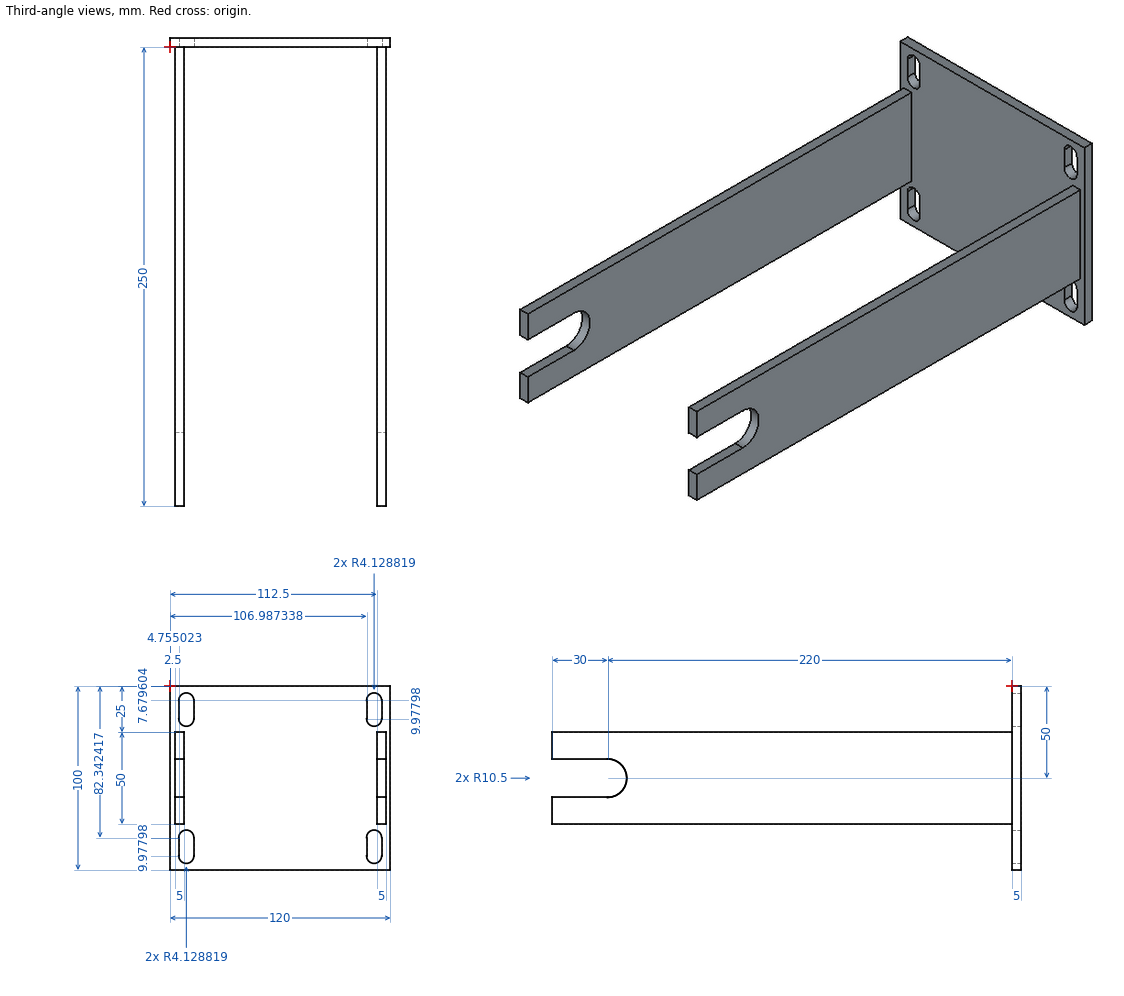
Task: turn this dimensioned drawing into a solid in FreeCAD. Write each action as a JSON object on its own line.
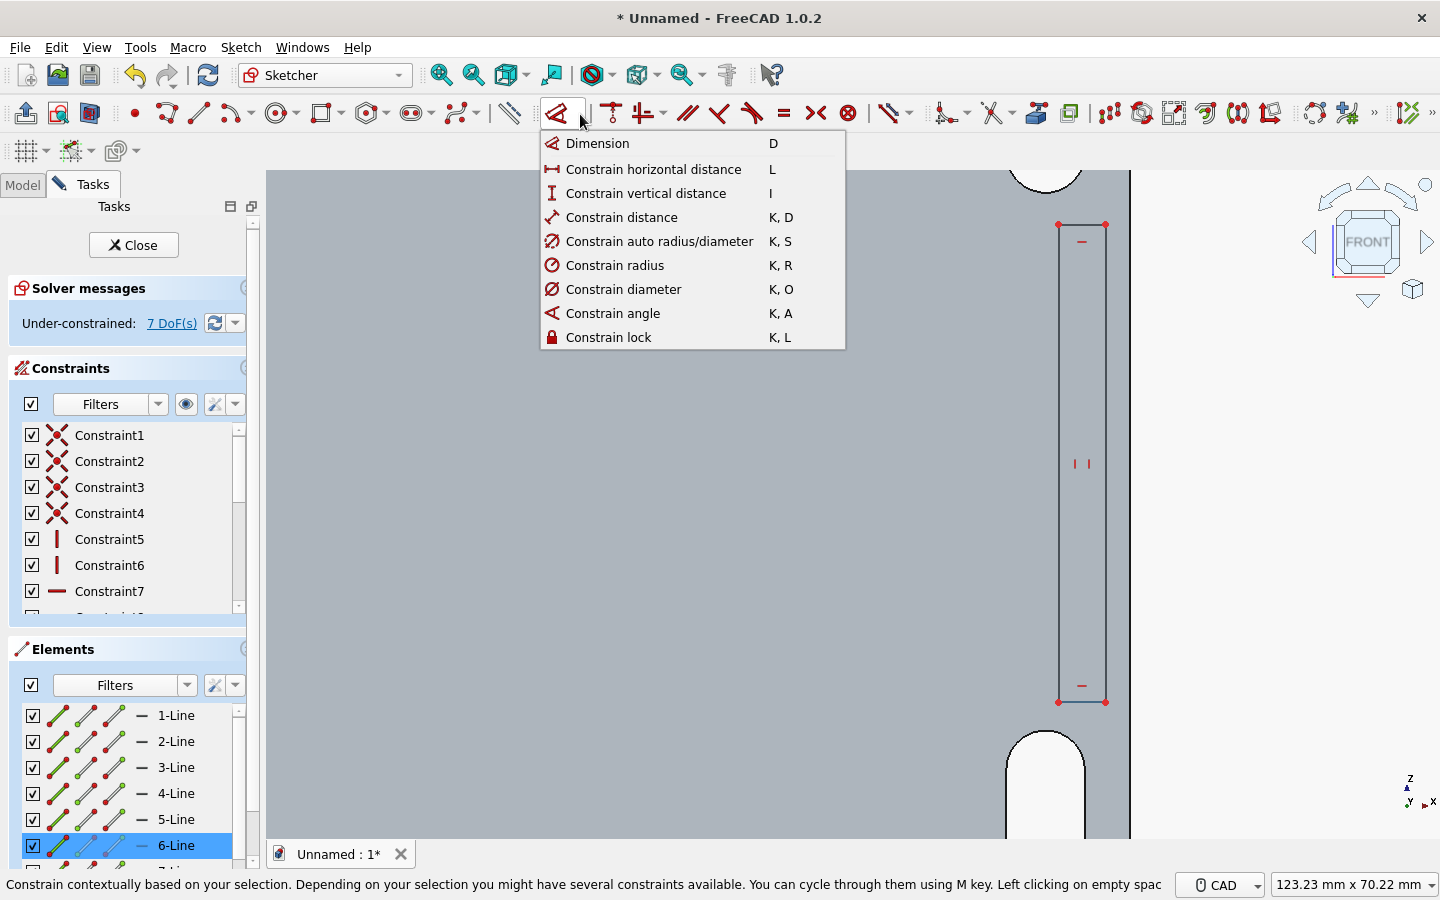
{"action": "left_click", "coordinate": [693, 169]}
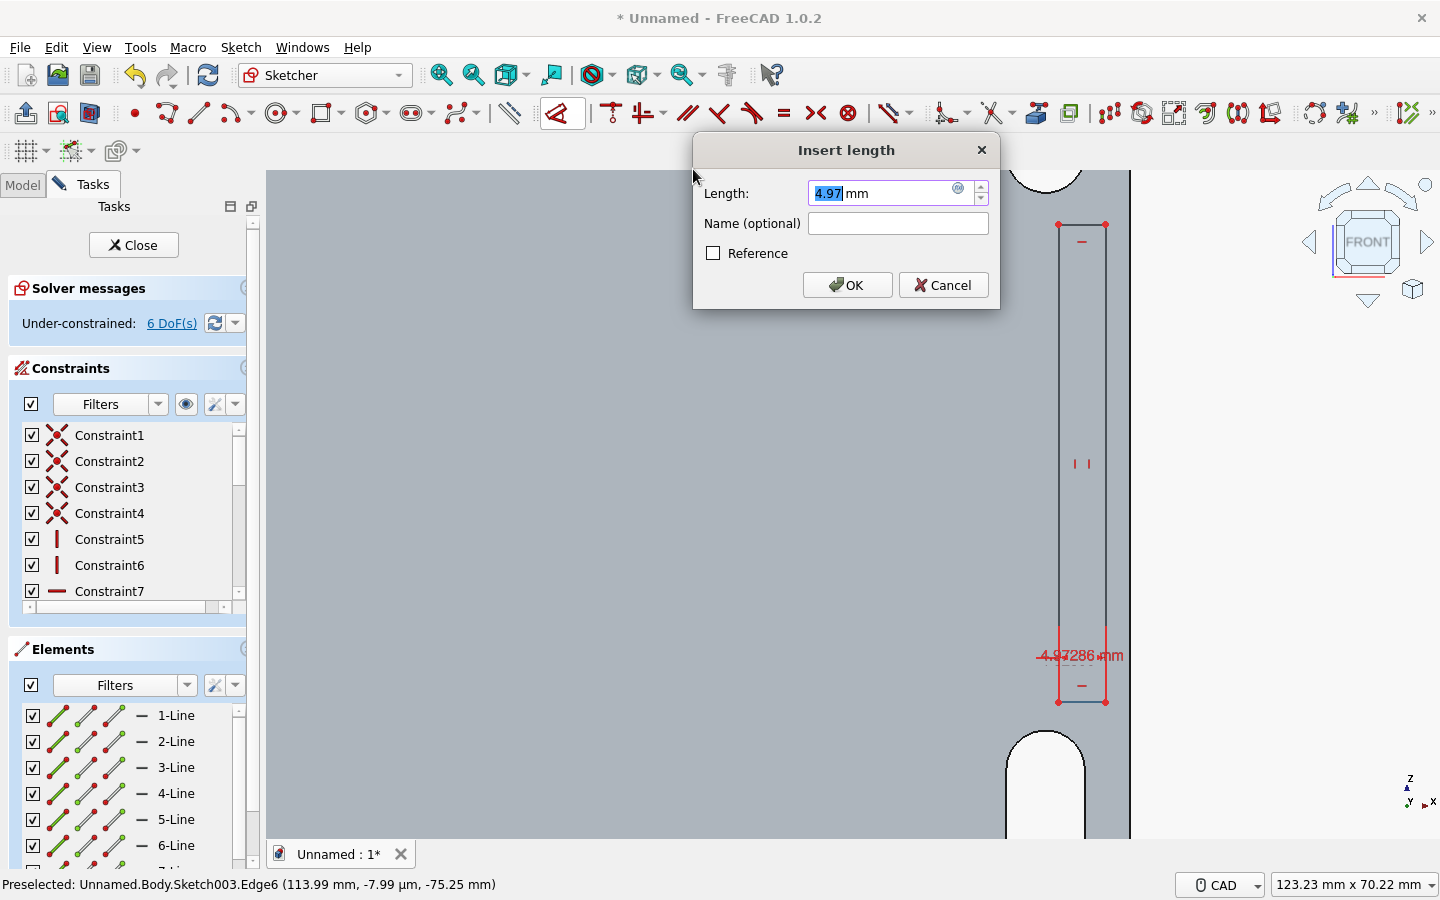
{"action": "type", "text": "5"}
{"action": "key", "text": "Return"}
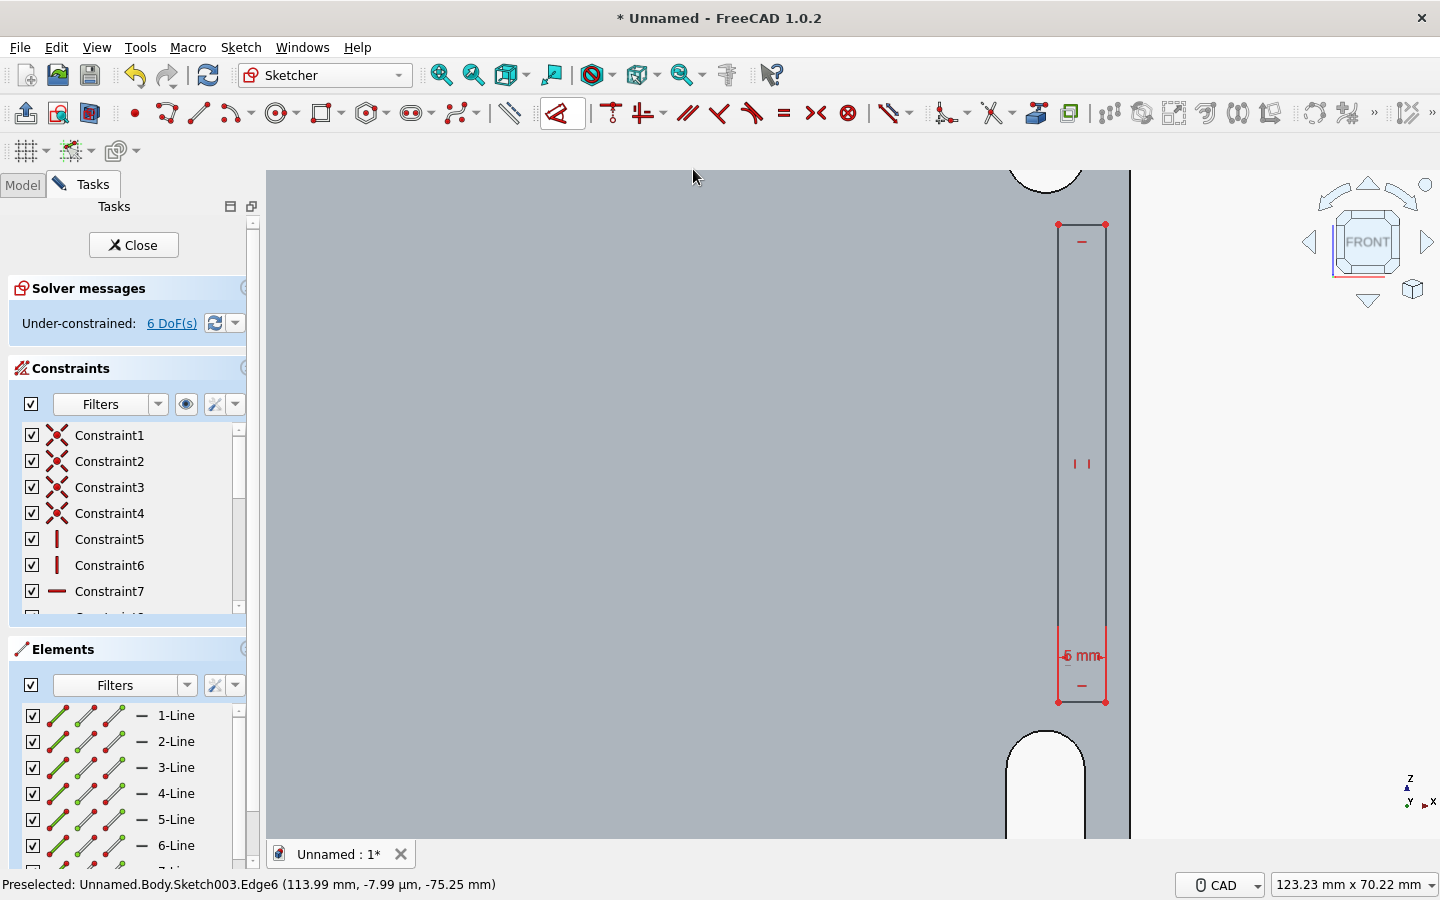
{"action": "scroll", "coordinate": [1074, 702], "scroll_direction": "down", "scroll_amount": 3}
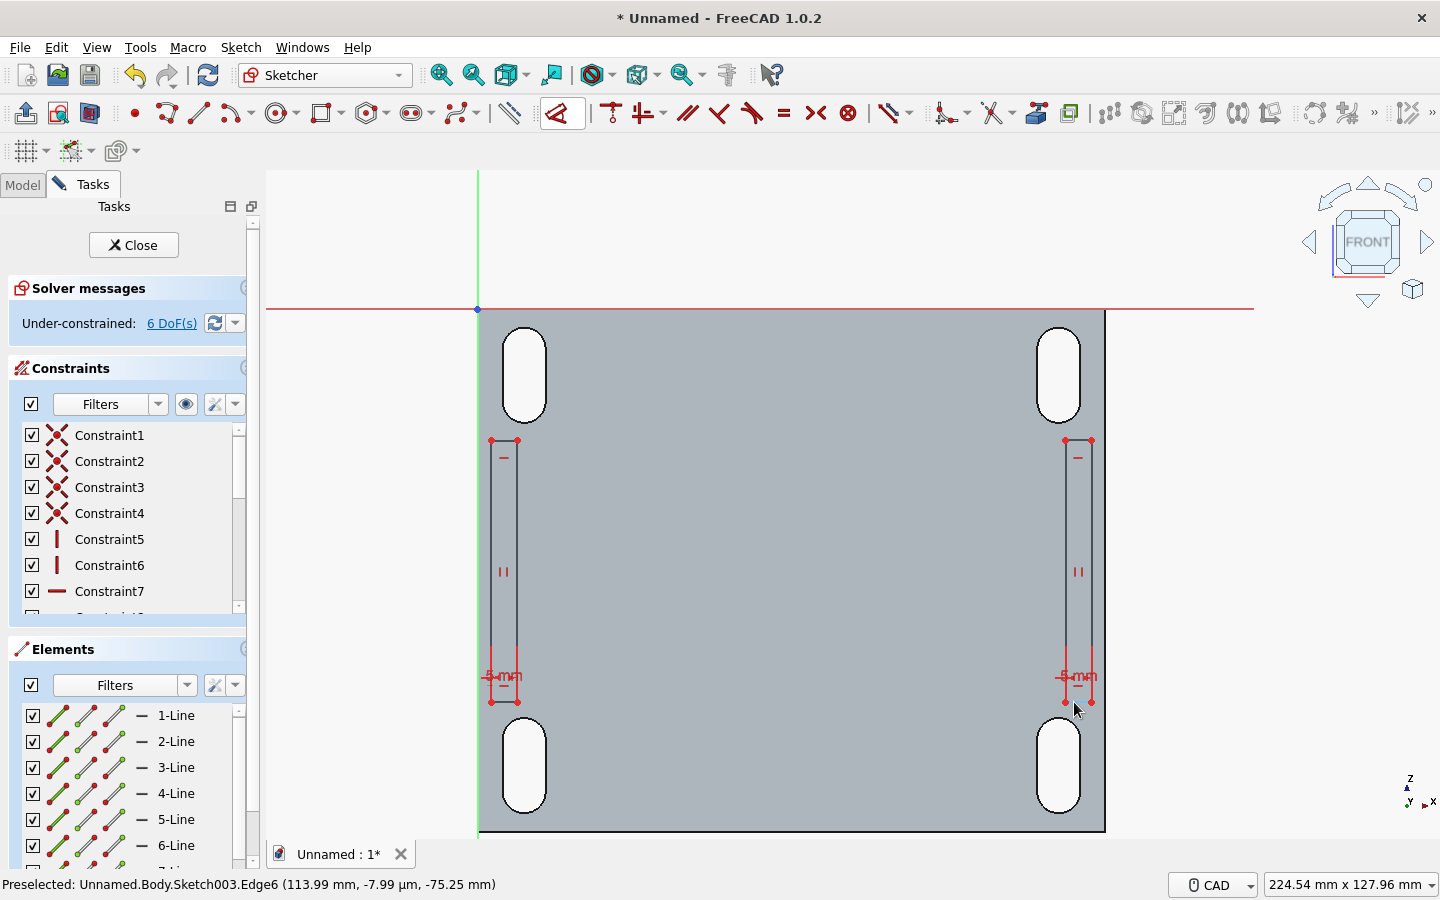
{"action": "left_click", "coordinate": [491, 519]}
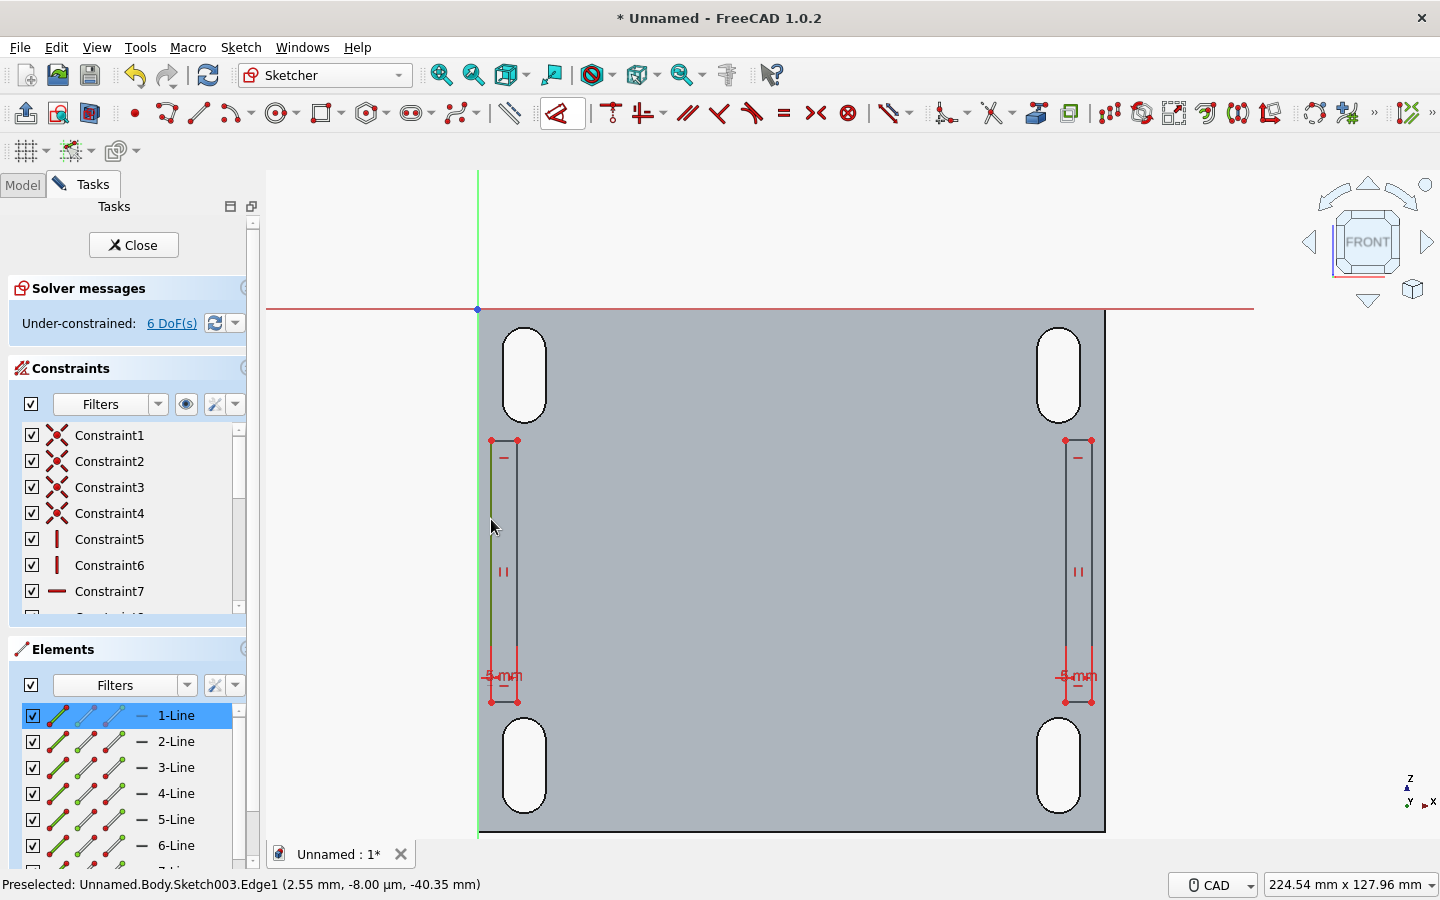
{"action": "key", "text": "i"}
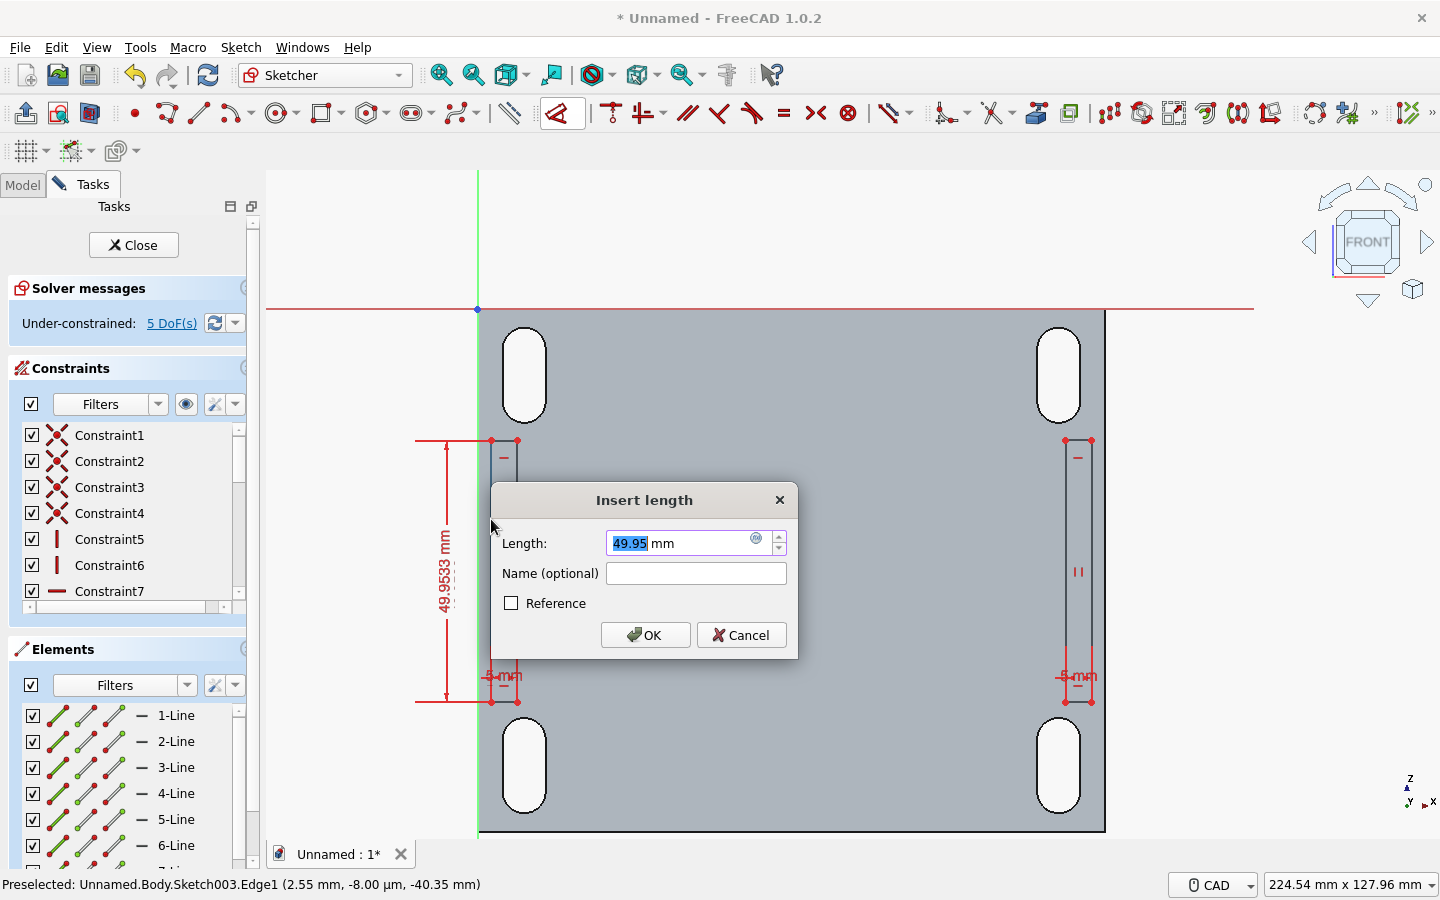
{"action": "type", "text": "50"}
{"action": "key", "text": "Return"}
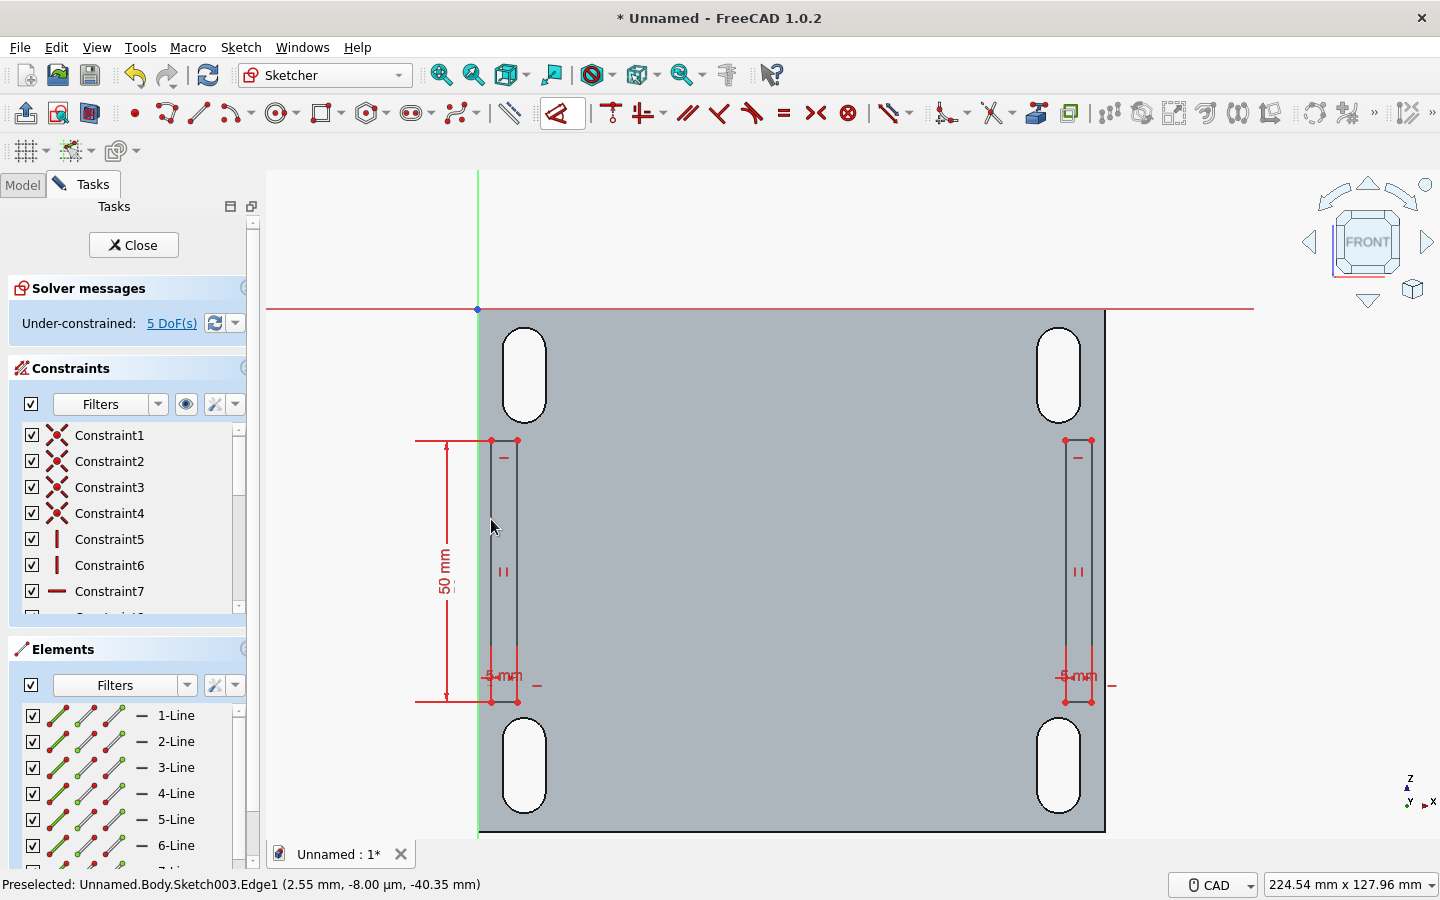
{"action": "left_click", "coordinate": [1066, 519]}